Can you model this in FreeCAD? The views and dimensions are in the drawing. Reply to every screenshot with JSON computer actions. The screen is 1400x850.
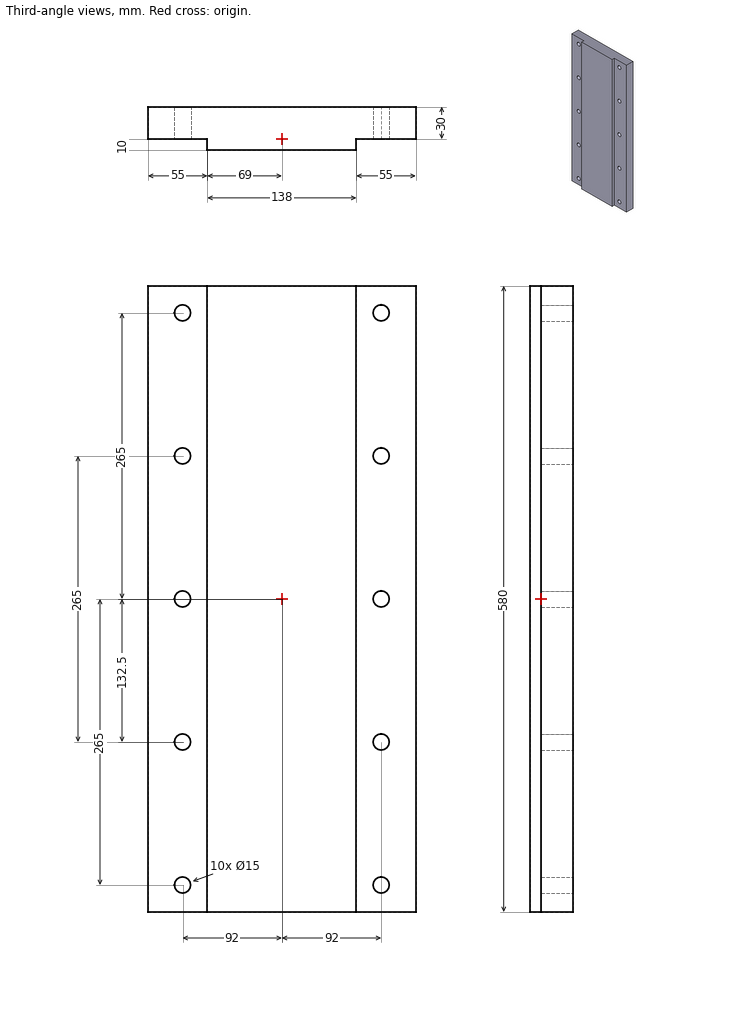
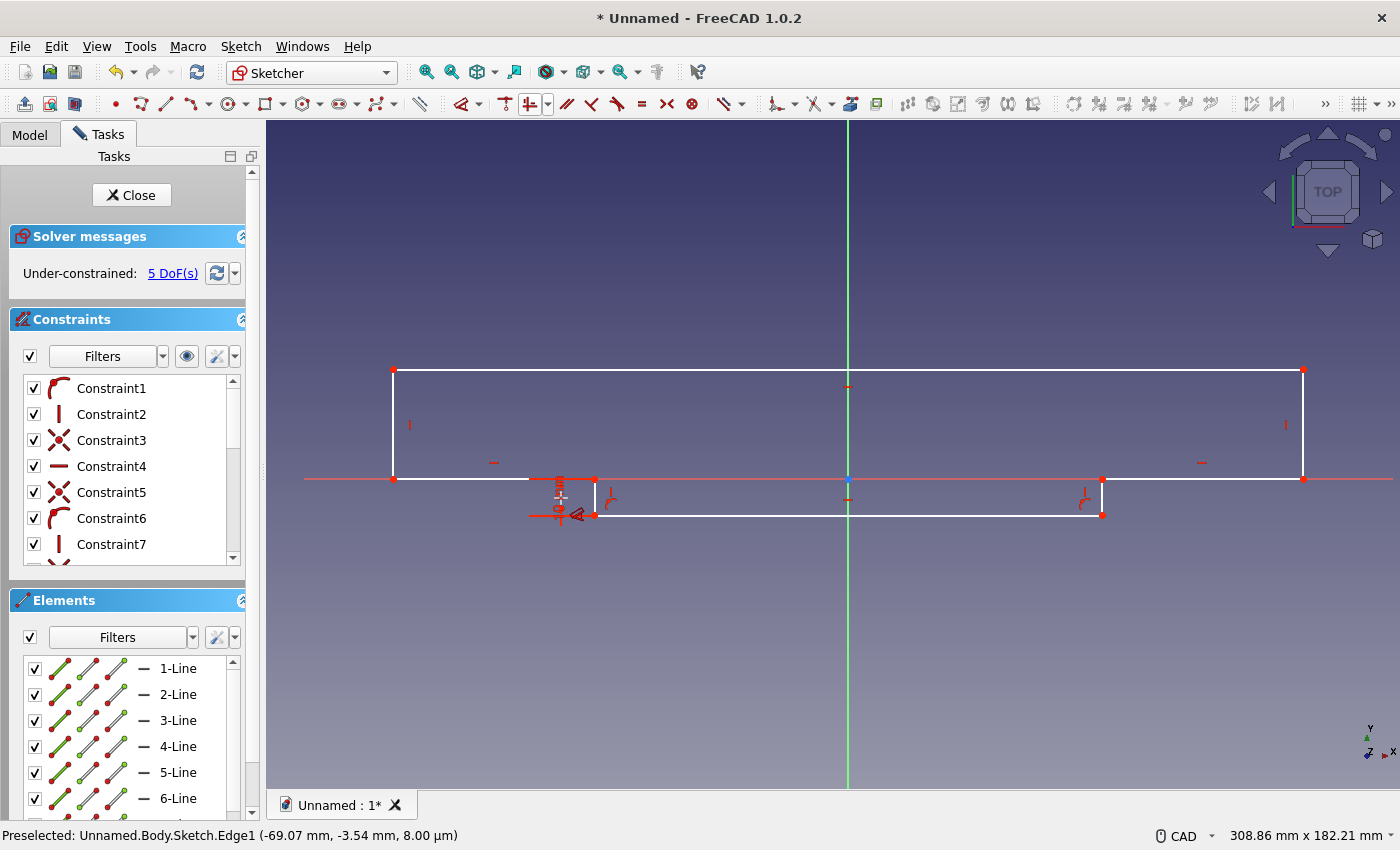
{"action": "left_click", "coordinate": [1162, 479]}
{"action": "left_click", "coordinate": [1169, 513]}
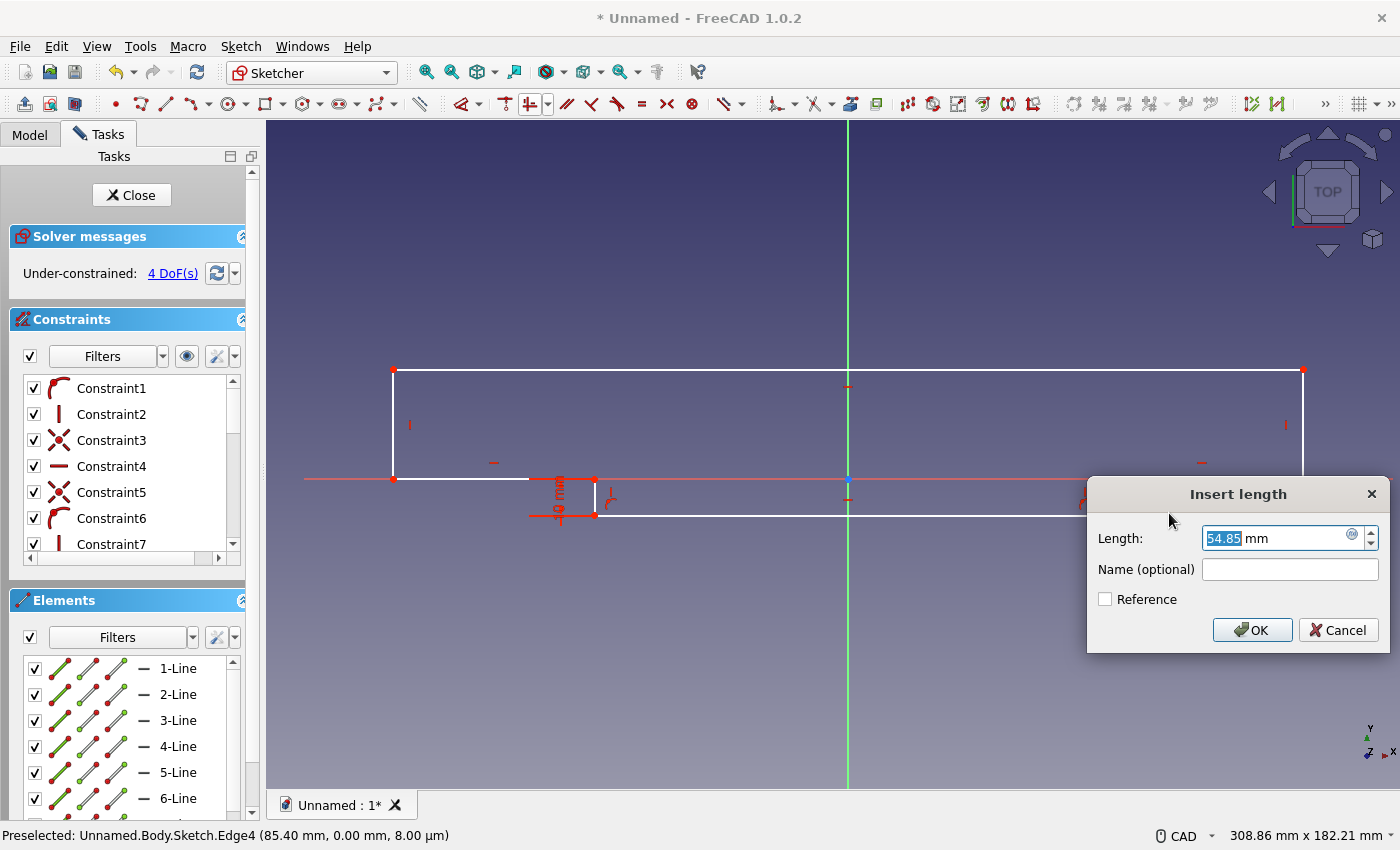
{"action": "type", "text": "55"}
{"action": "key", "text": "Return"}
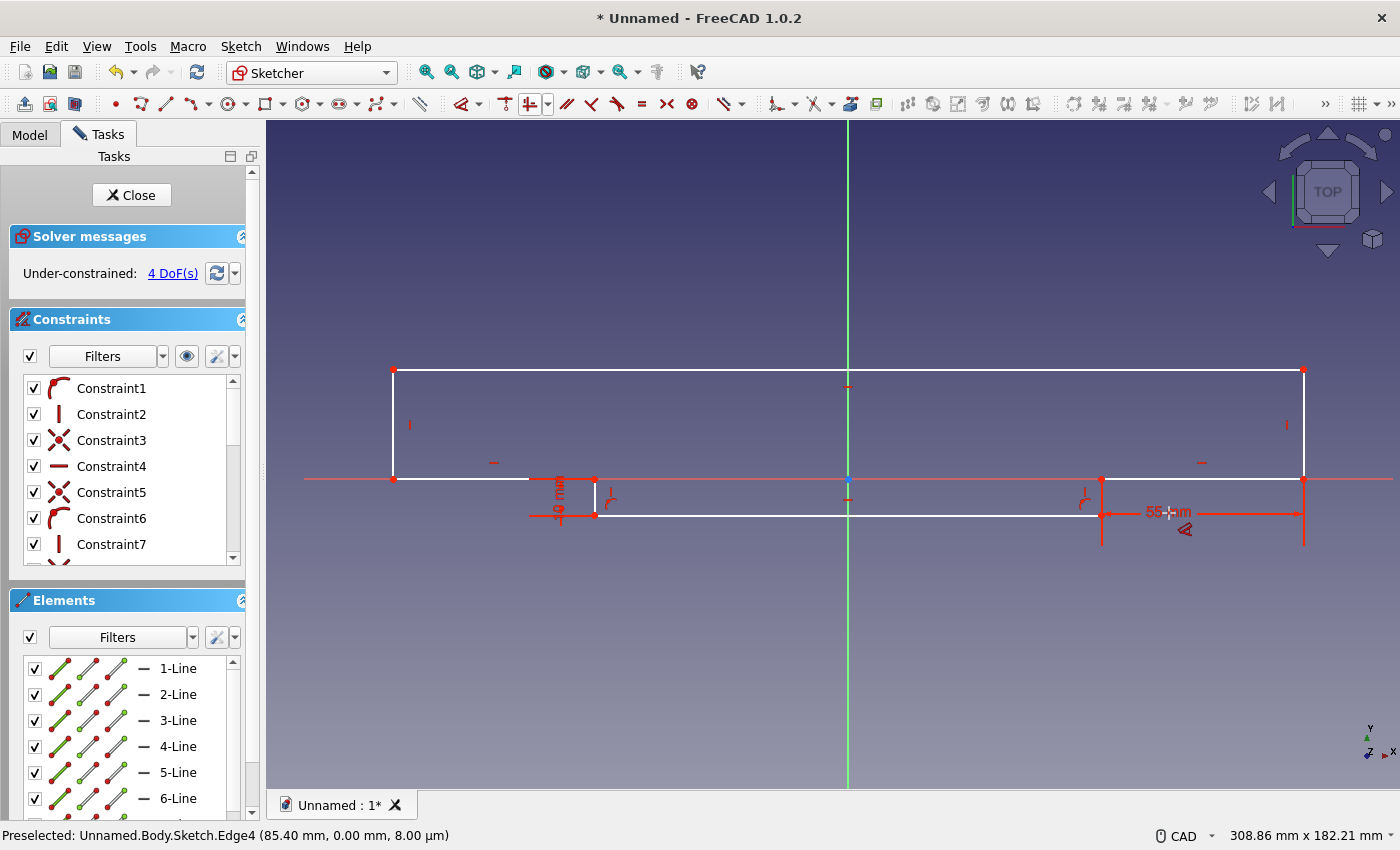
{"action": "scroll", "coordinate": [594, 479], "scroll_direction": "down", "scroll_amount": 2}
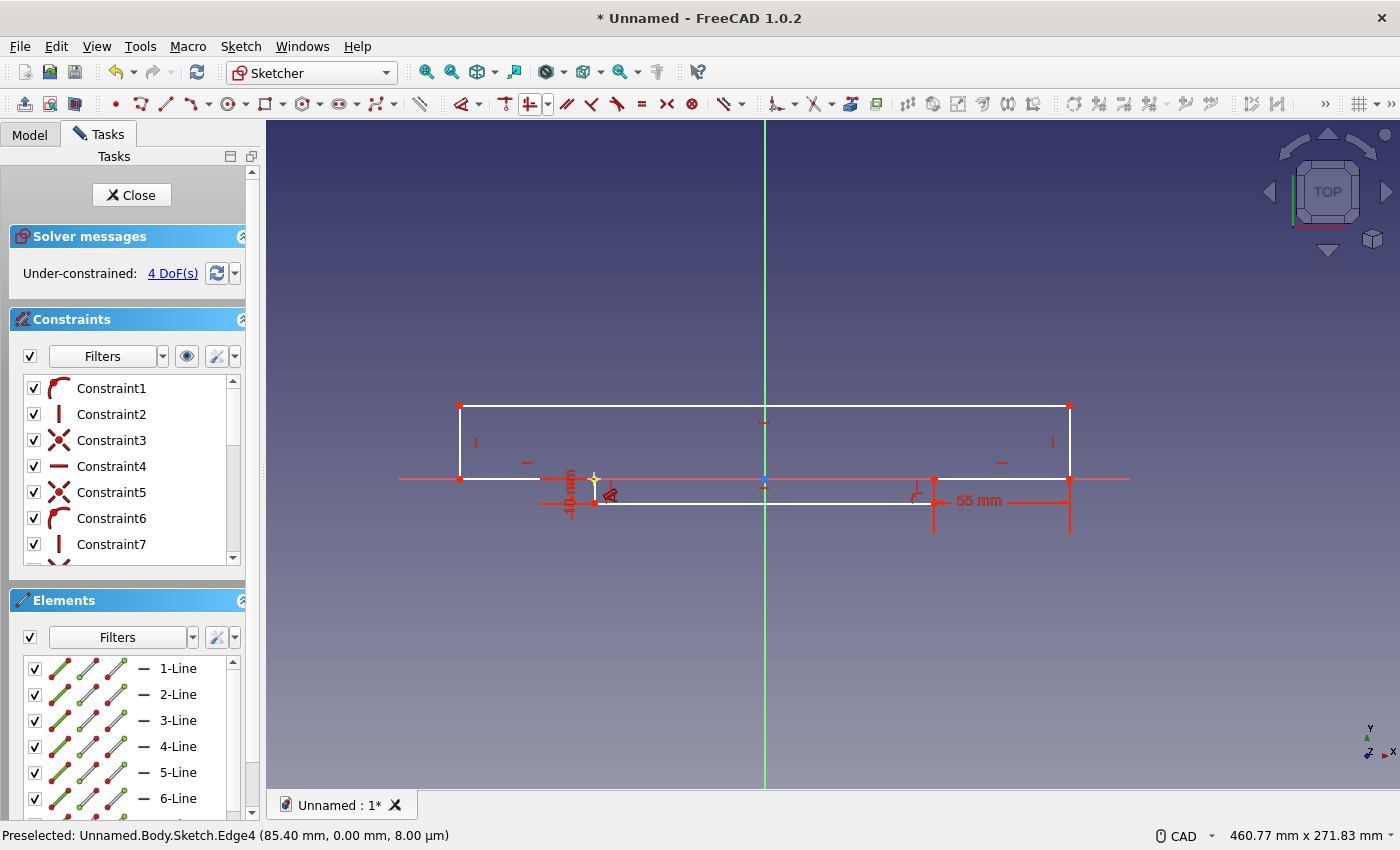
{"action": "left_click", "coordinate": [1070, 457]}
{"action": "left_click", "coordinate": [1104, 443]}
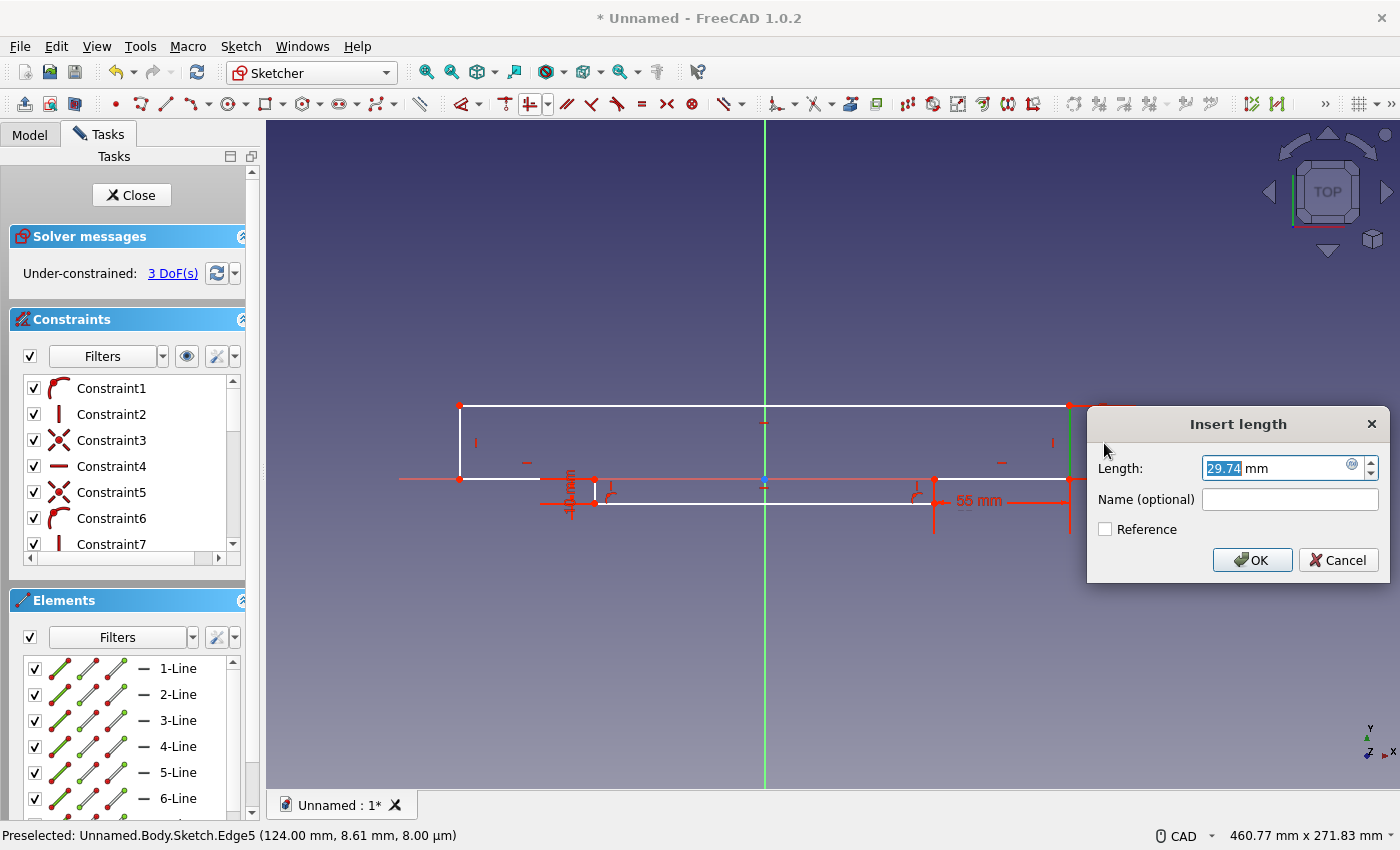
{"action": "type", "text": "30"}
{"action": "key", "text": "Return"}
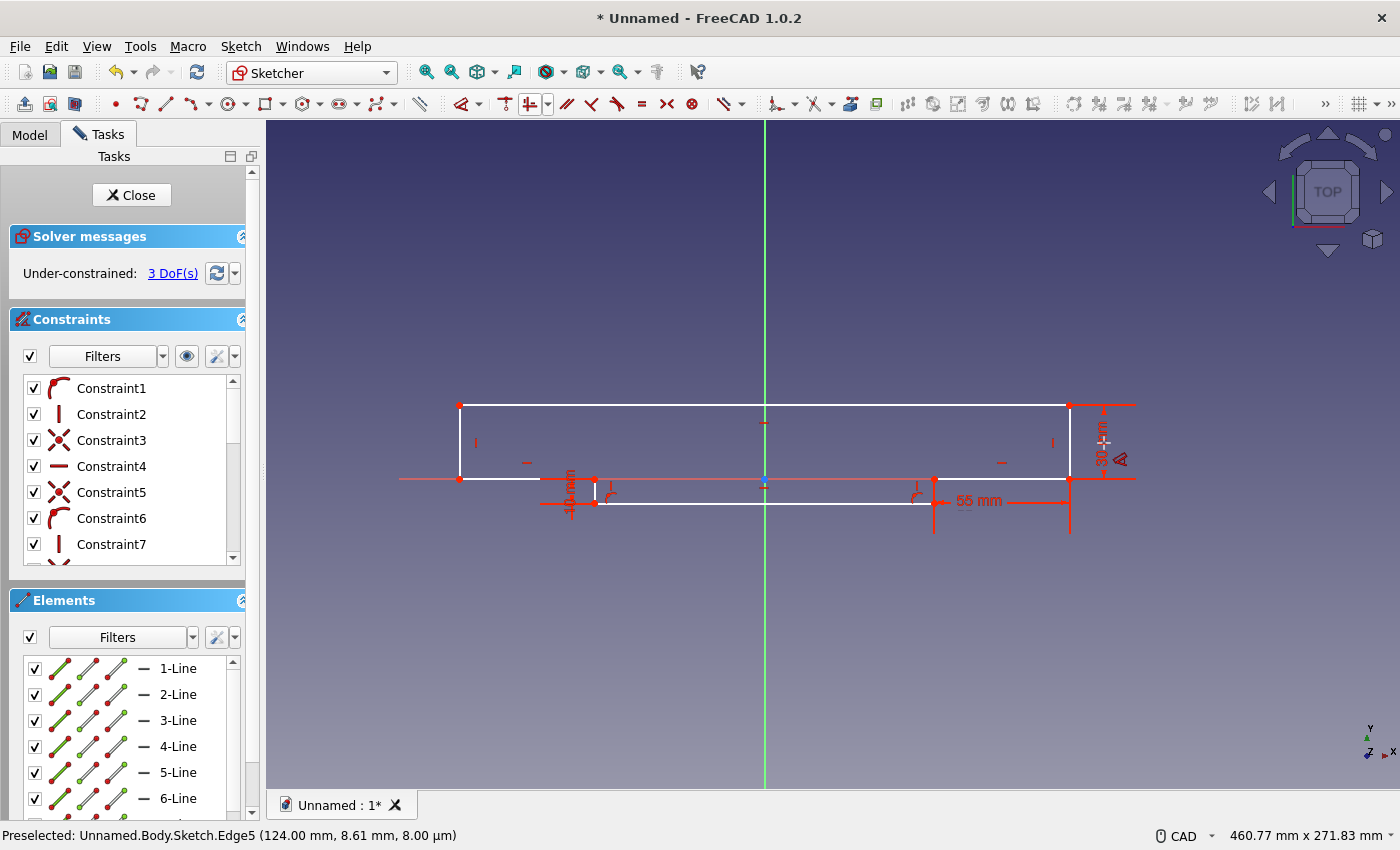
{"action": "left_click", "coordinate": [500, 479]}
{"action": "left_click", "coordinate": [527, 513]}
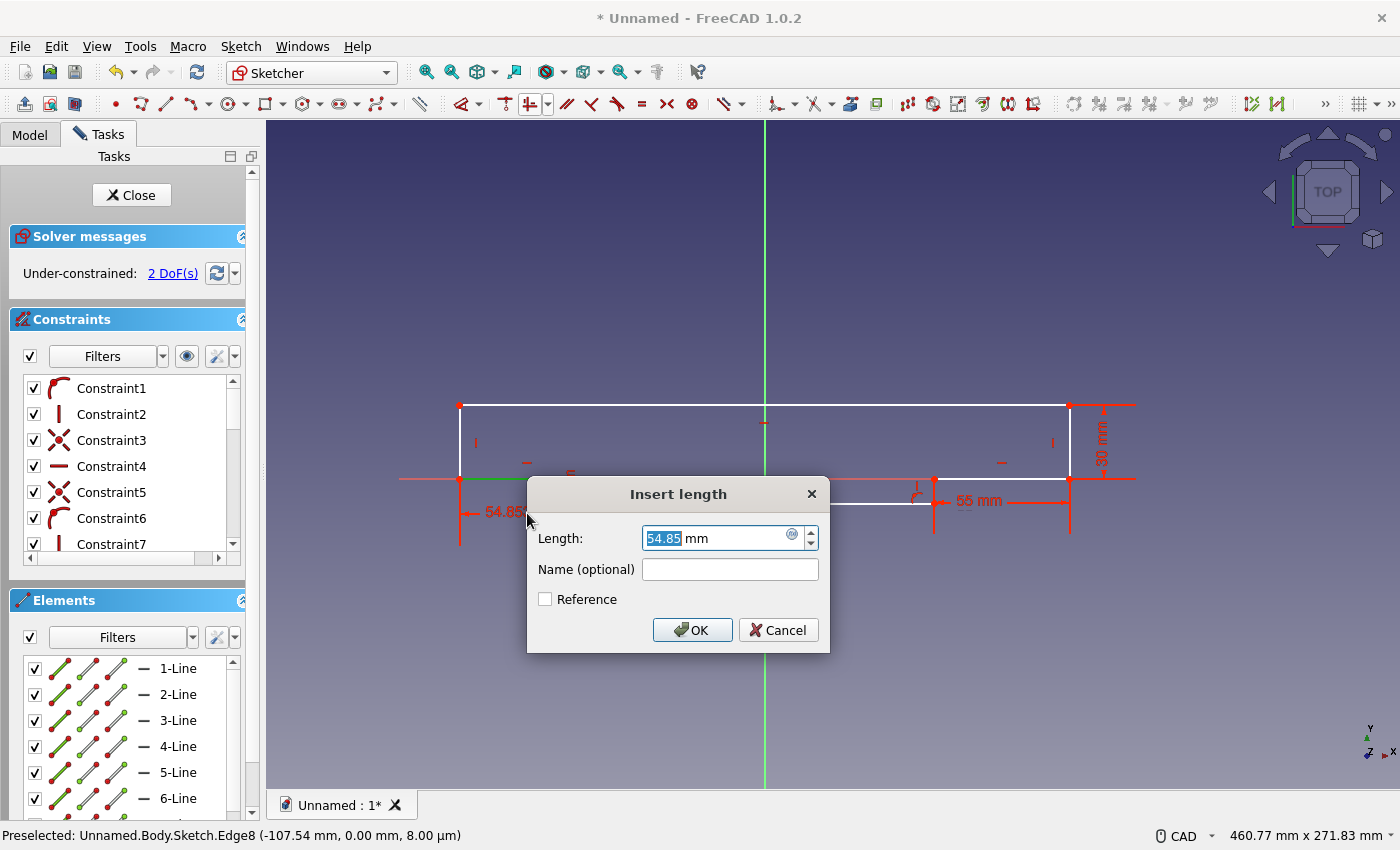
{"action": "type", "text": "55"}
{"action": "key", "text": "Return"}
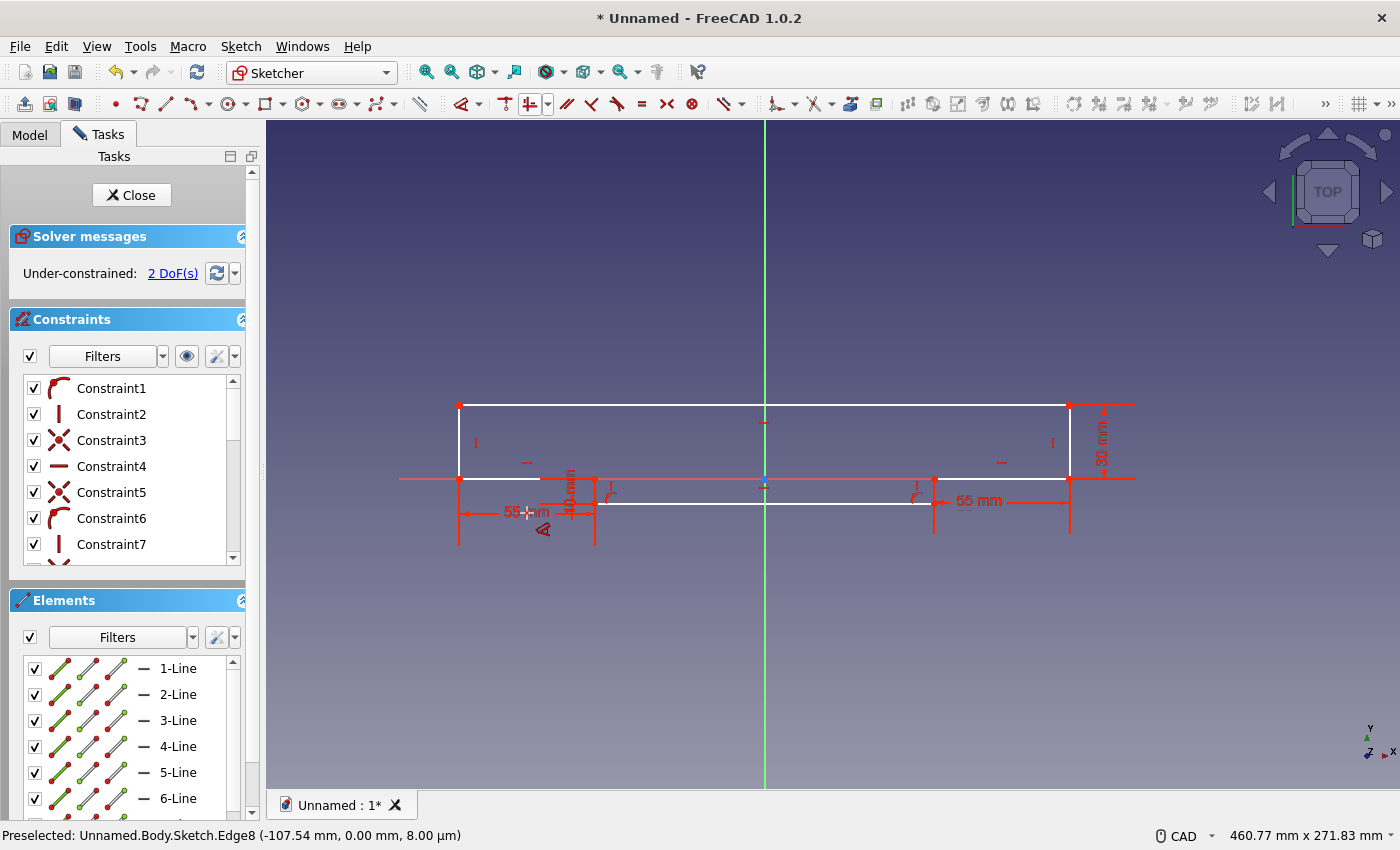
{"action": "left_click", "coordinate": [697, 504]}
{"action": "left_click", "coordinate": [687, 538]}